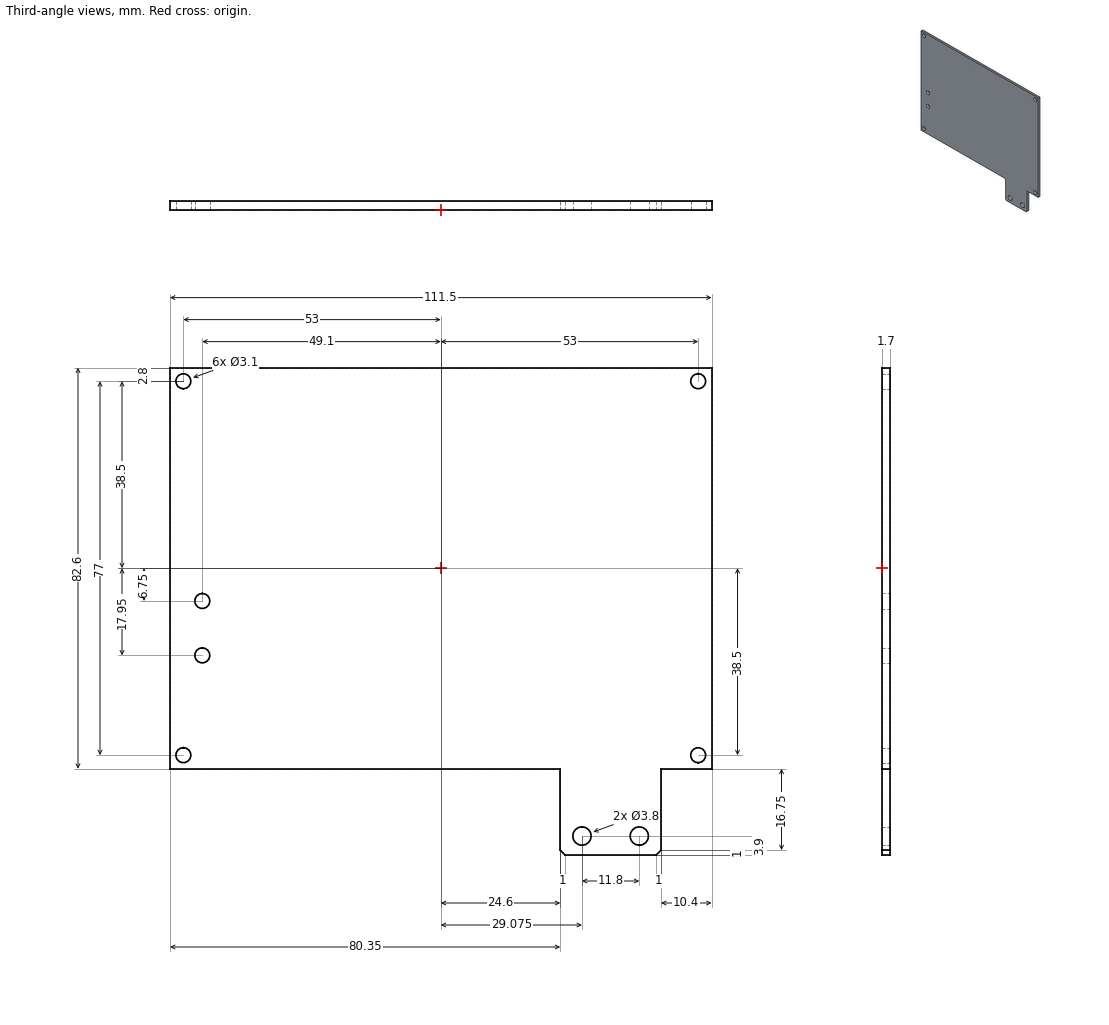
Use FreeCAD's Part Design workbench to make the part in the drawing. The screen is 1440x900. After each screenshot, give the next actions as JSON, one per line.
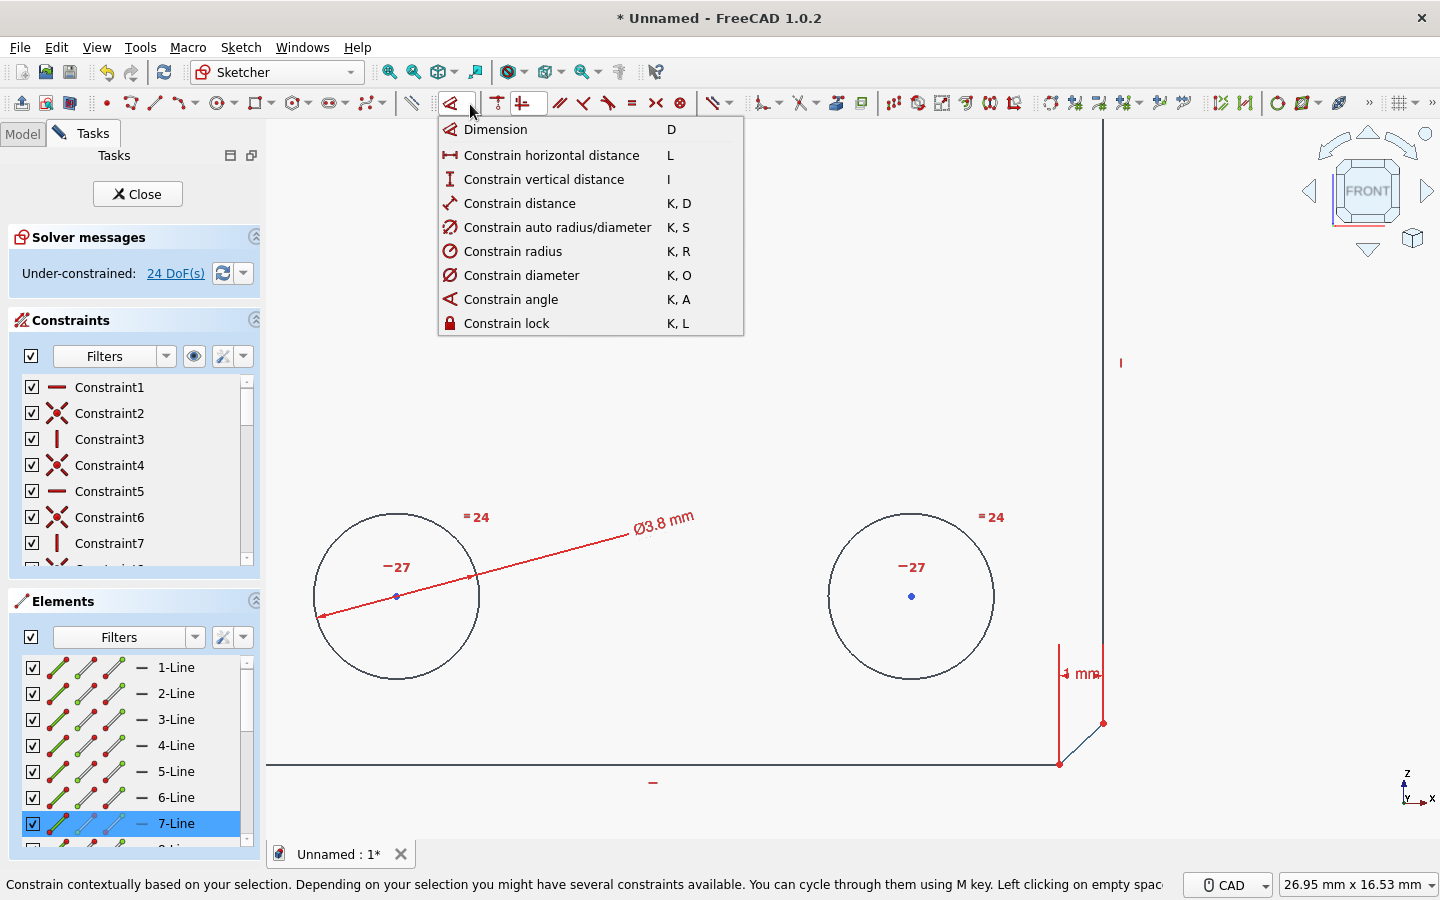
{"action": "left_click", "coordinate": [591, 179]}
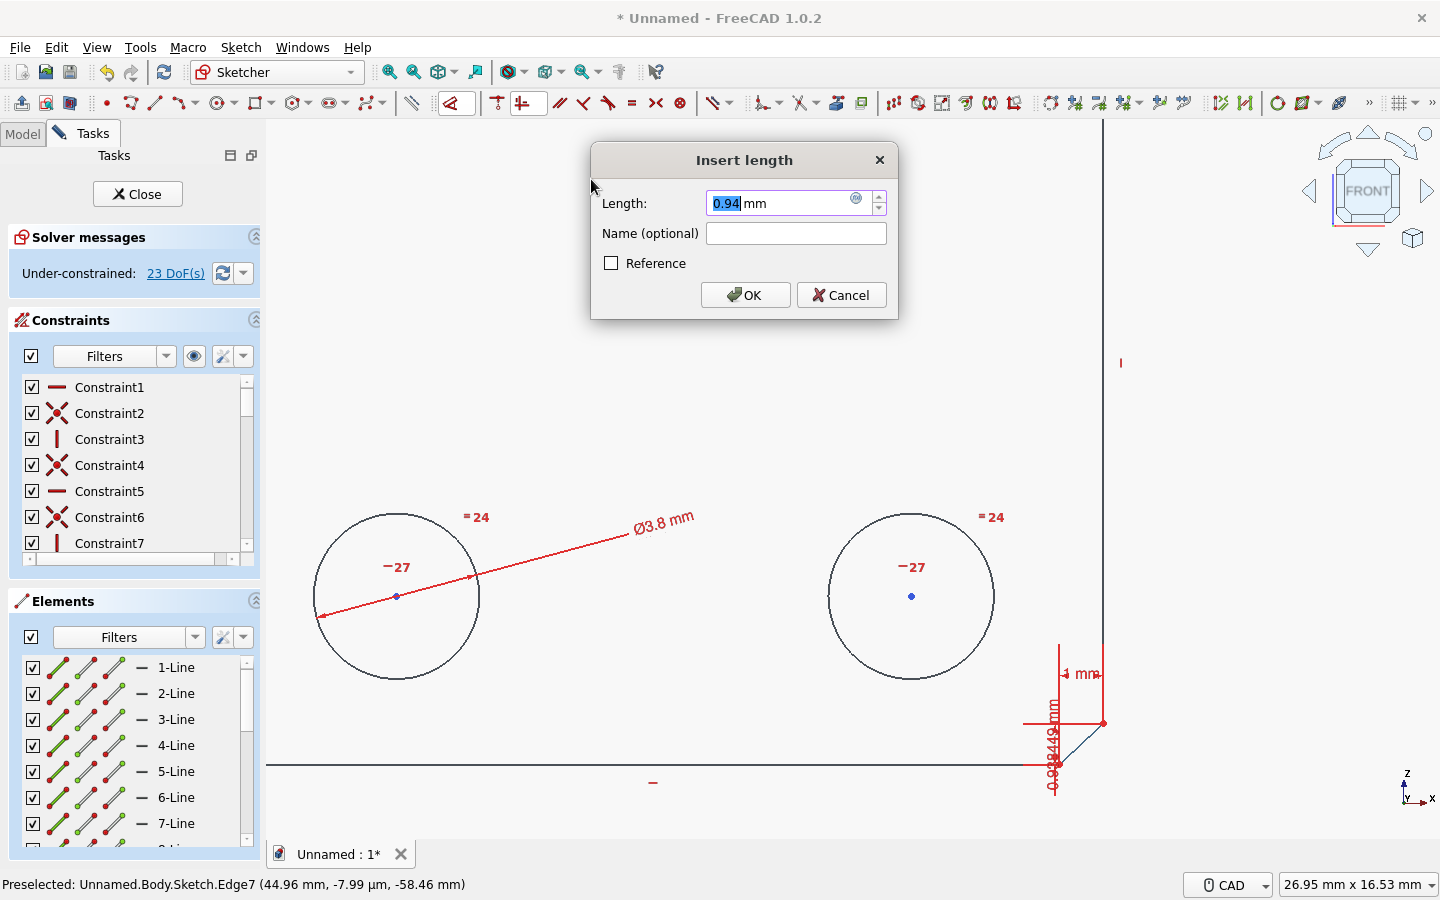
{"action": "type", "text": "1"}
{"action": "key", "text": "Return"}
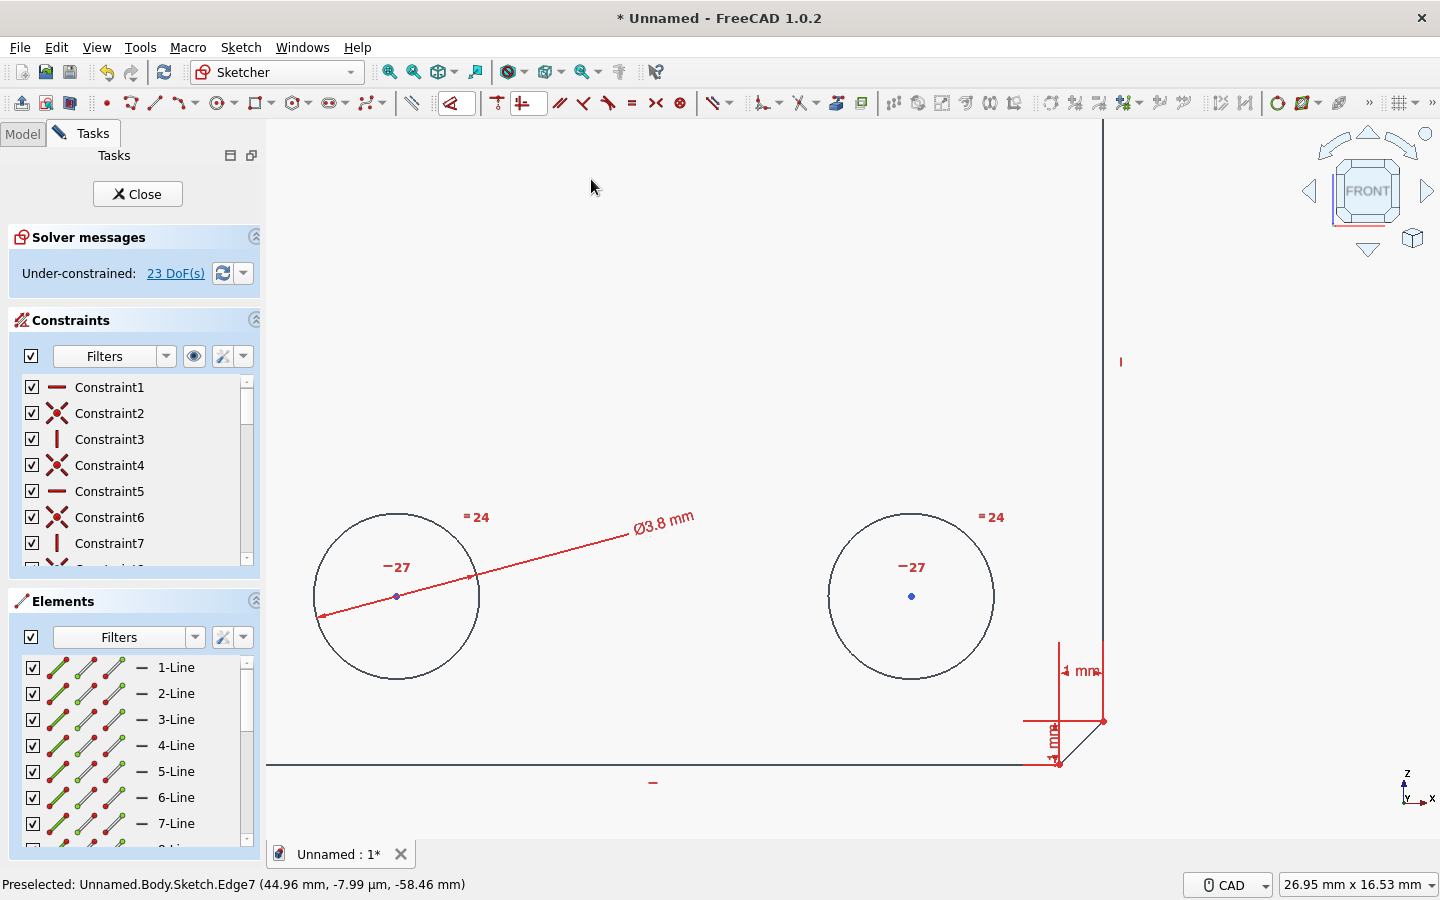
{"action": "scroll", "coordinate": [990, 716], "scroll_direction": "down", "scroll_amount": 11}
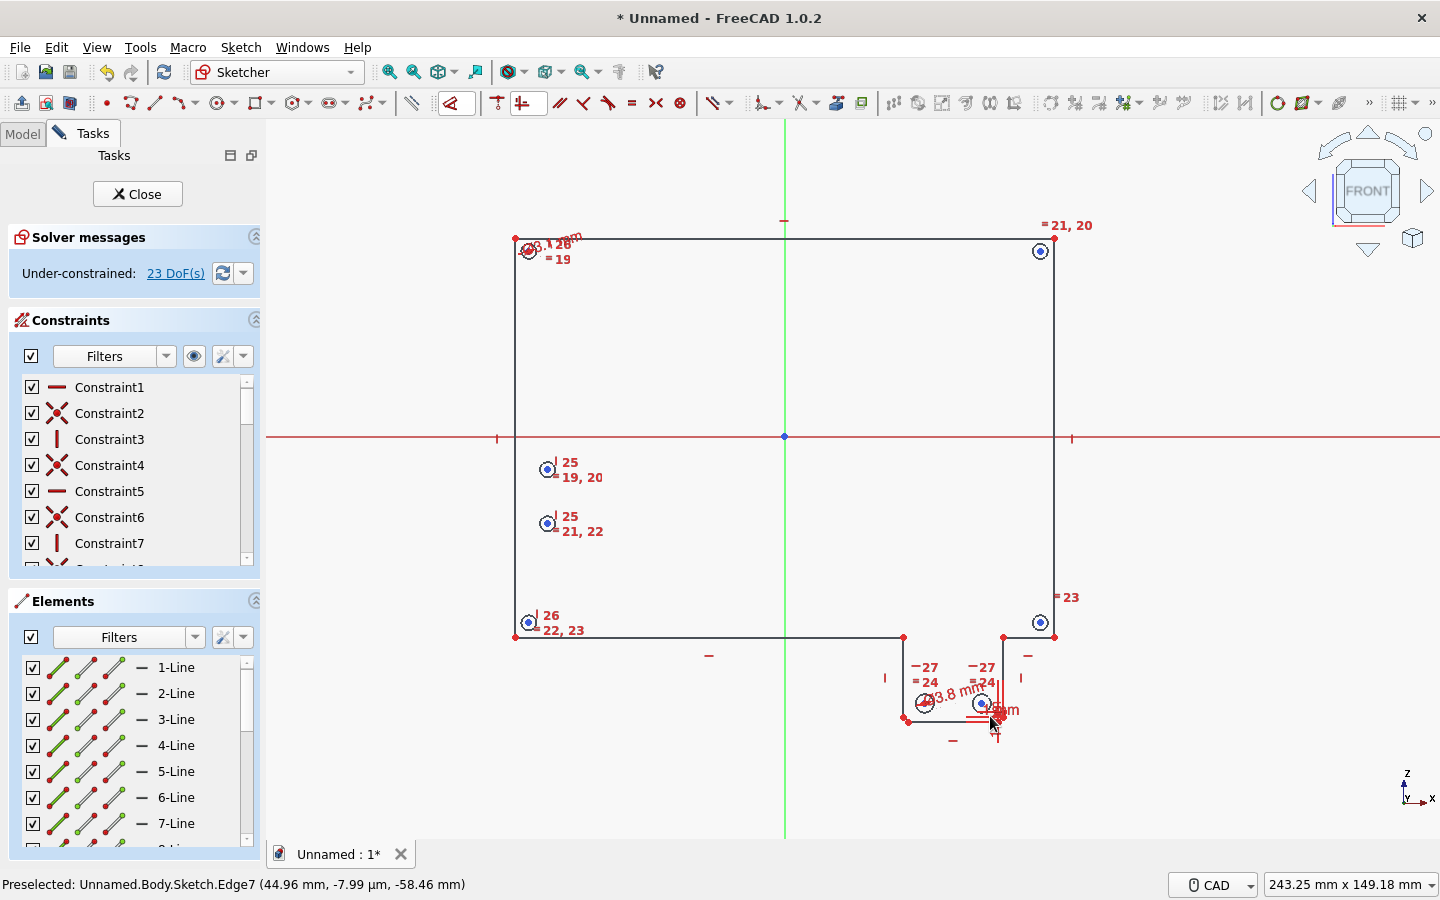
{"action": "scroll", "coordinate": [907, 721], "scroll_direction": "up", "scroll_amount": 11}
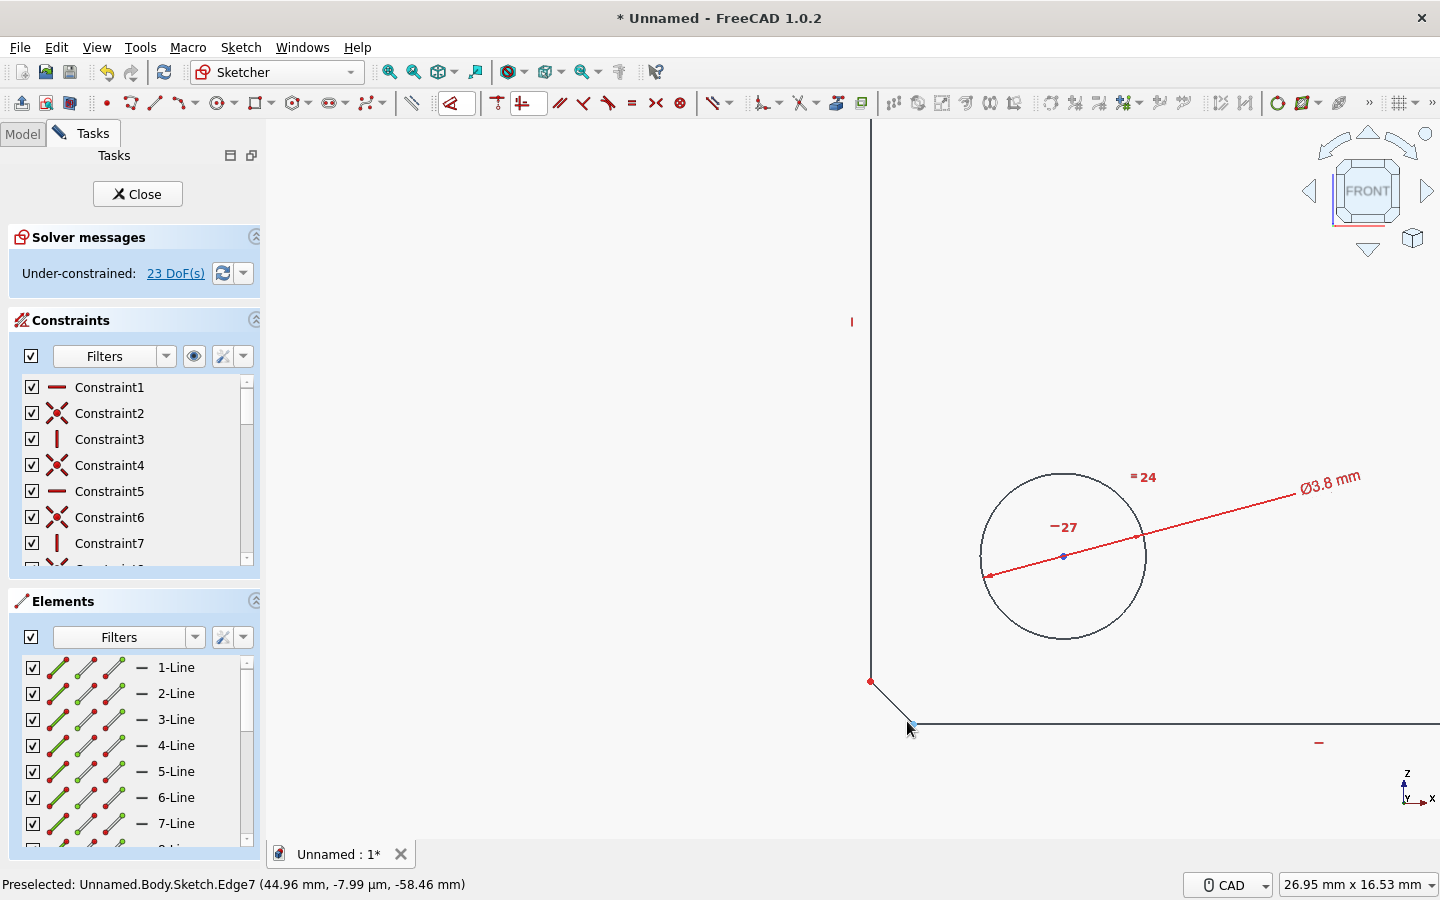
{"action": "left_click", "coordinate": [901, 712]}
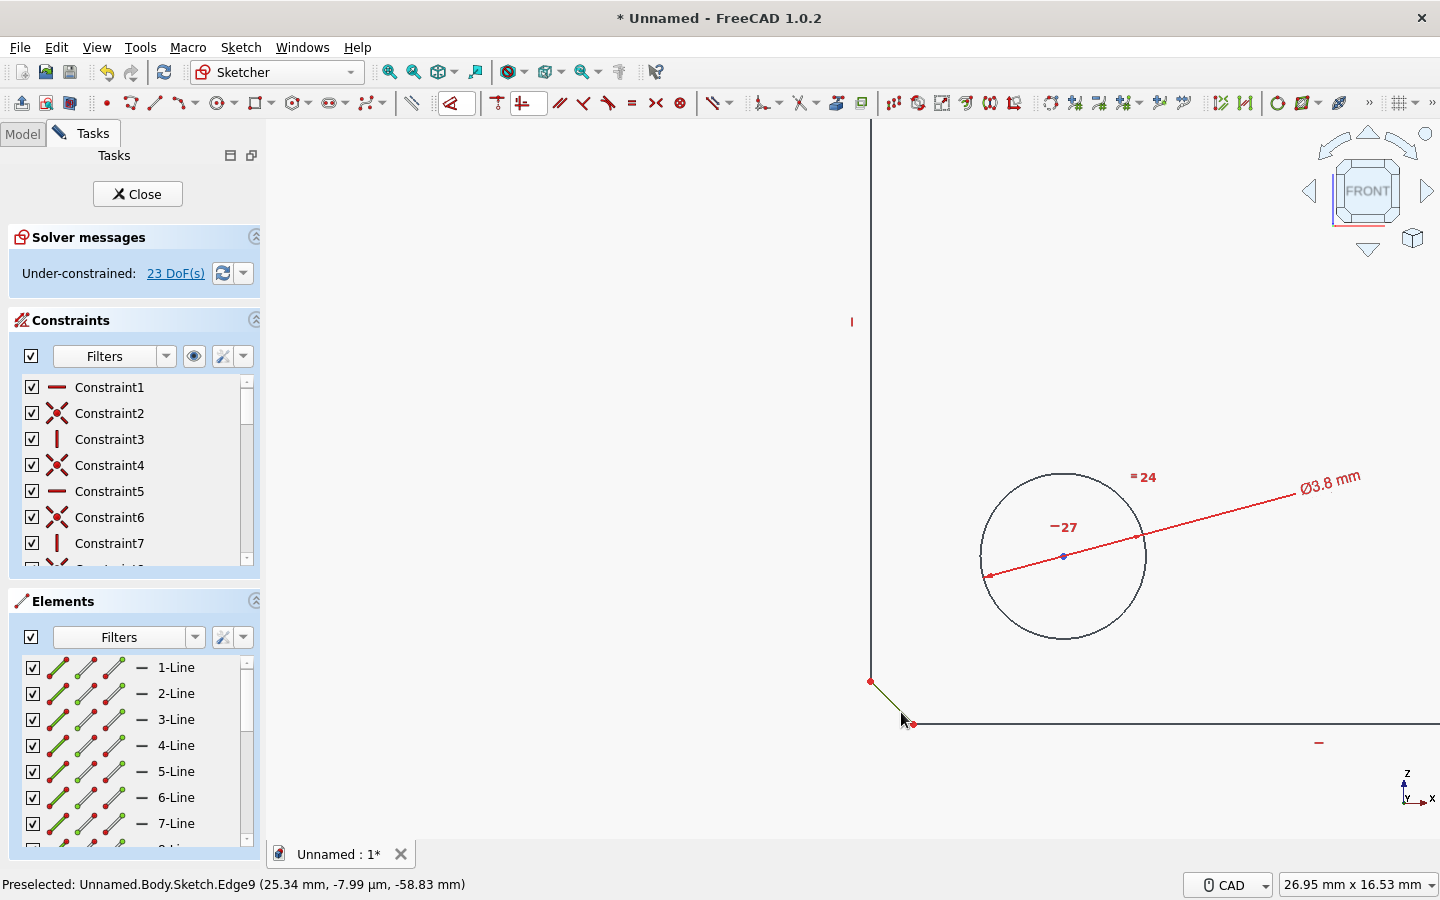
{"action": "left_click", "coordinate": [470, 104]}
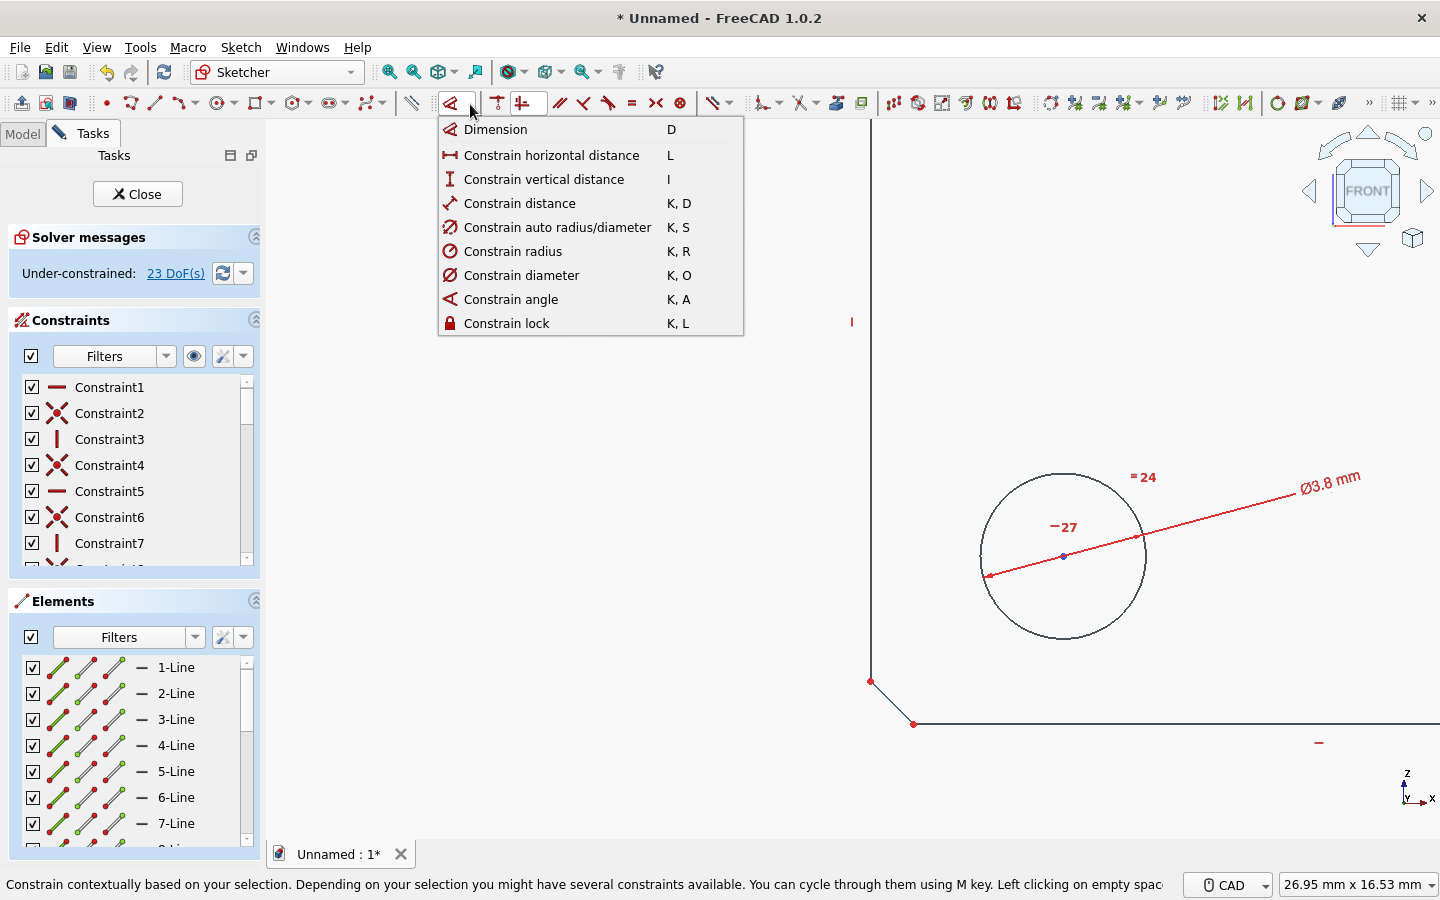
{"action": "left_click", "coordinate": [591, 155]}